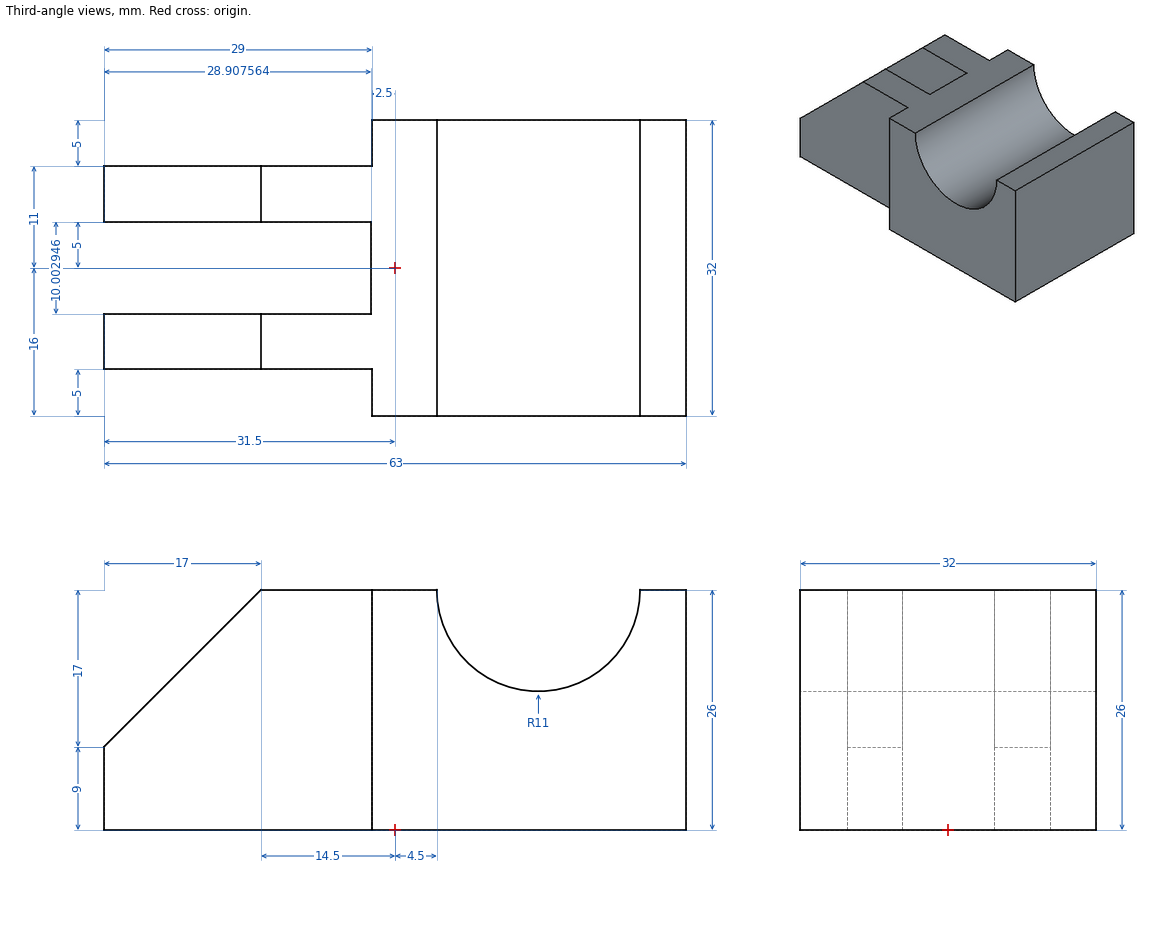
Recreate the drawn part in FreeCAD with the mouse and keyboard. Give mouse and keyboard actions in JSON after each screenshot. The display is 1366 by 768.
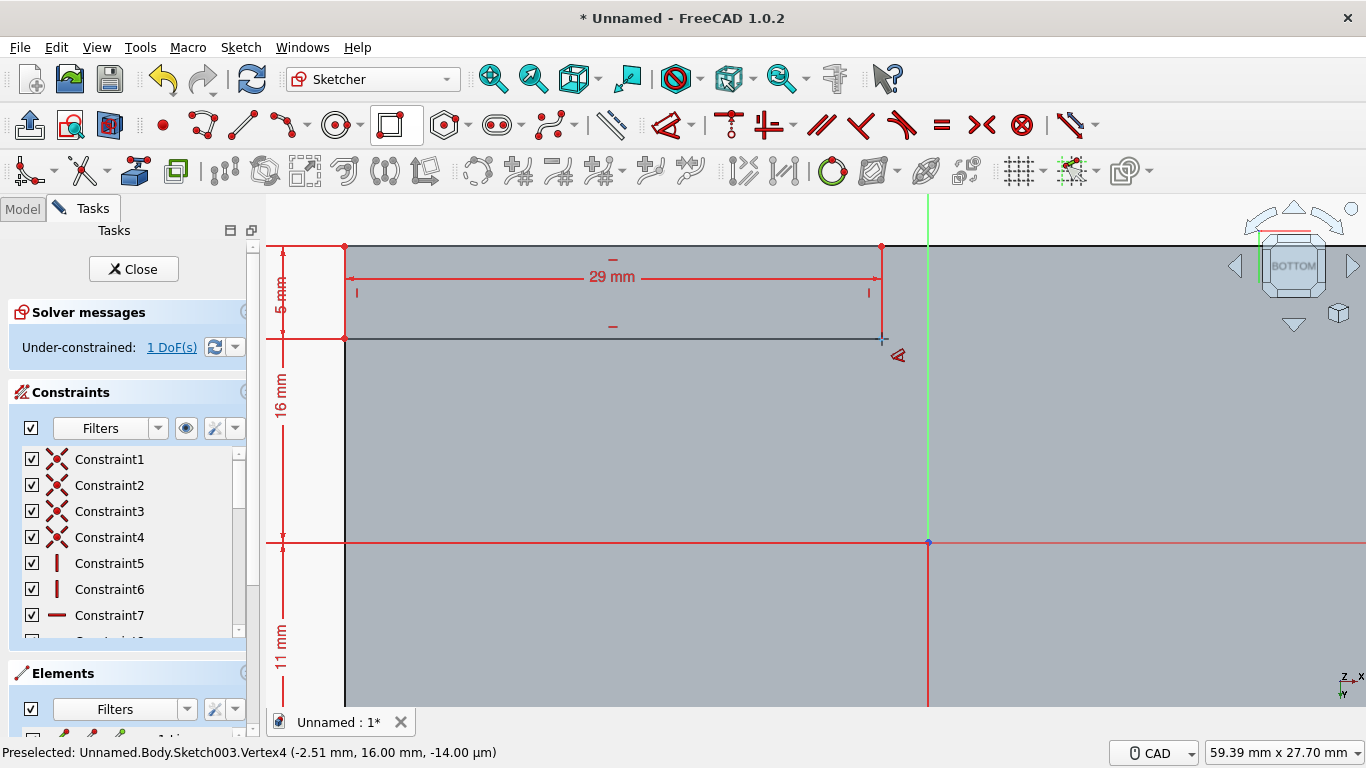
{"action": "left_click", "coordinate": [882, 339]}
{"action": "left_click", "coordinate": [905, 305]}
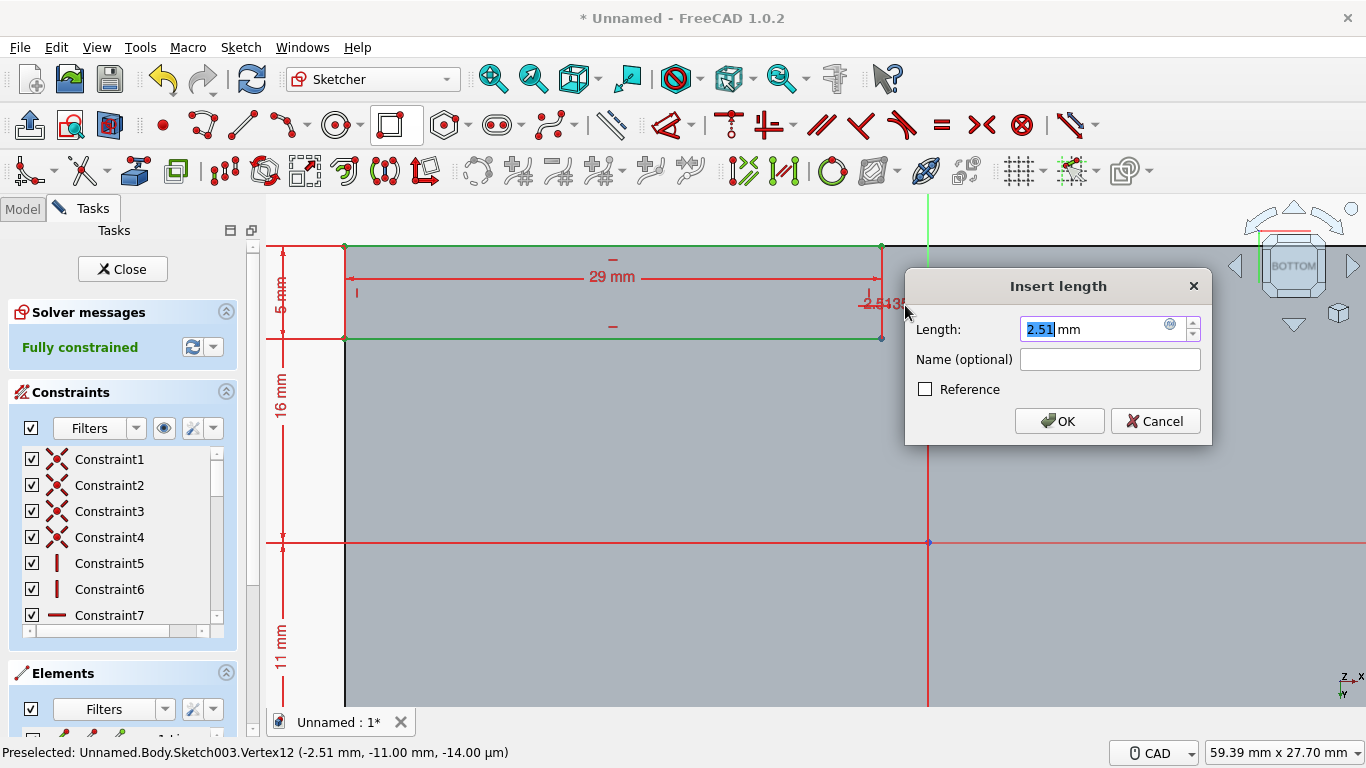
{"action": "type", "text": "2.5"}
{"action": "key", "text": "Return"}
{"action": "key", "text": "Escape"}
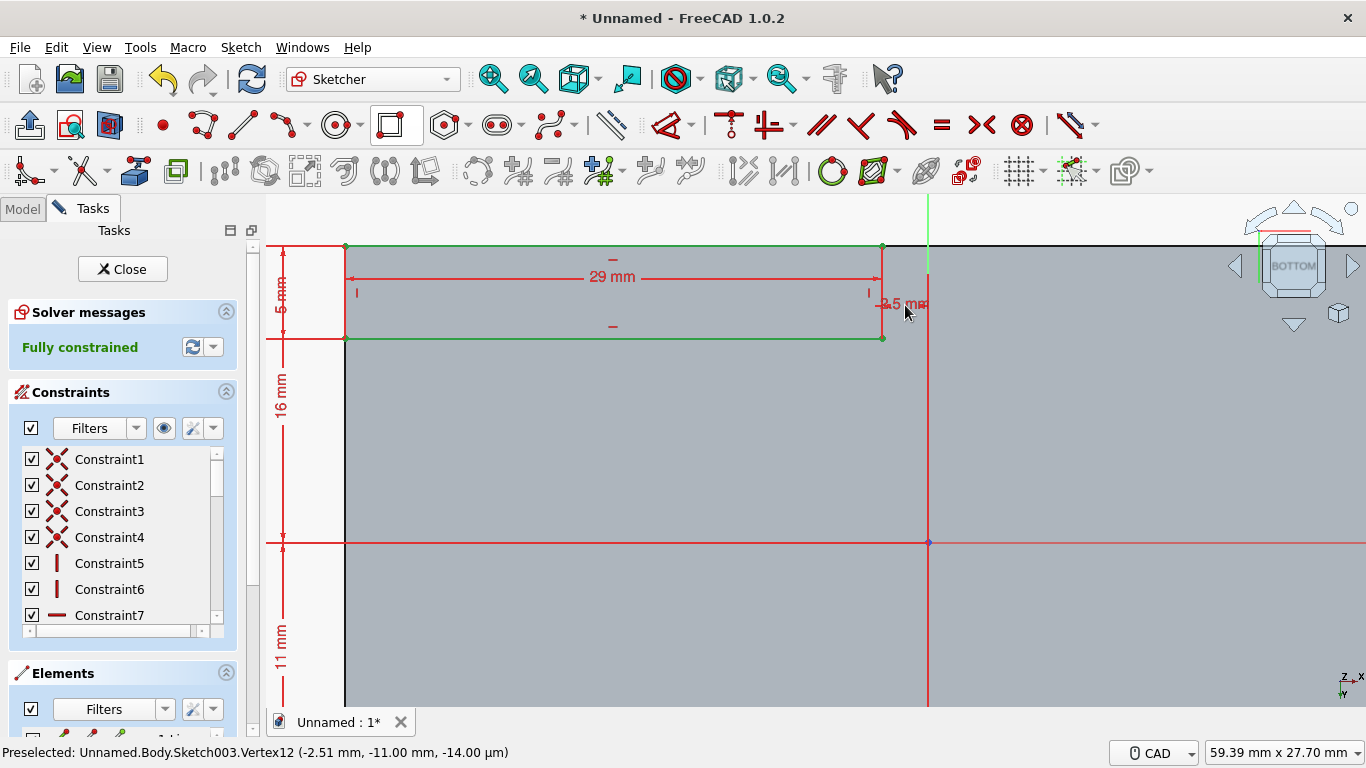
{"action": "left_click", "coordinate": [123, 269]}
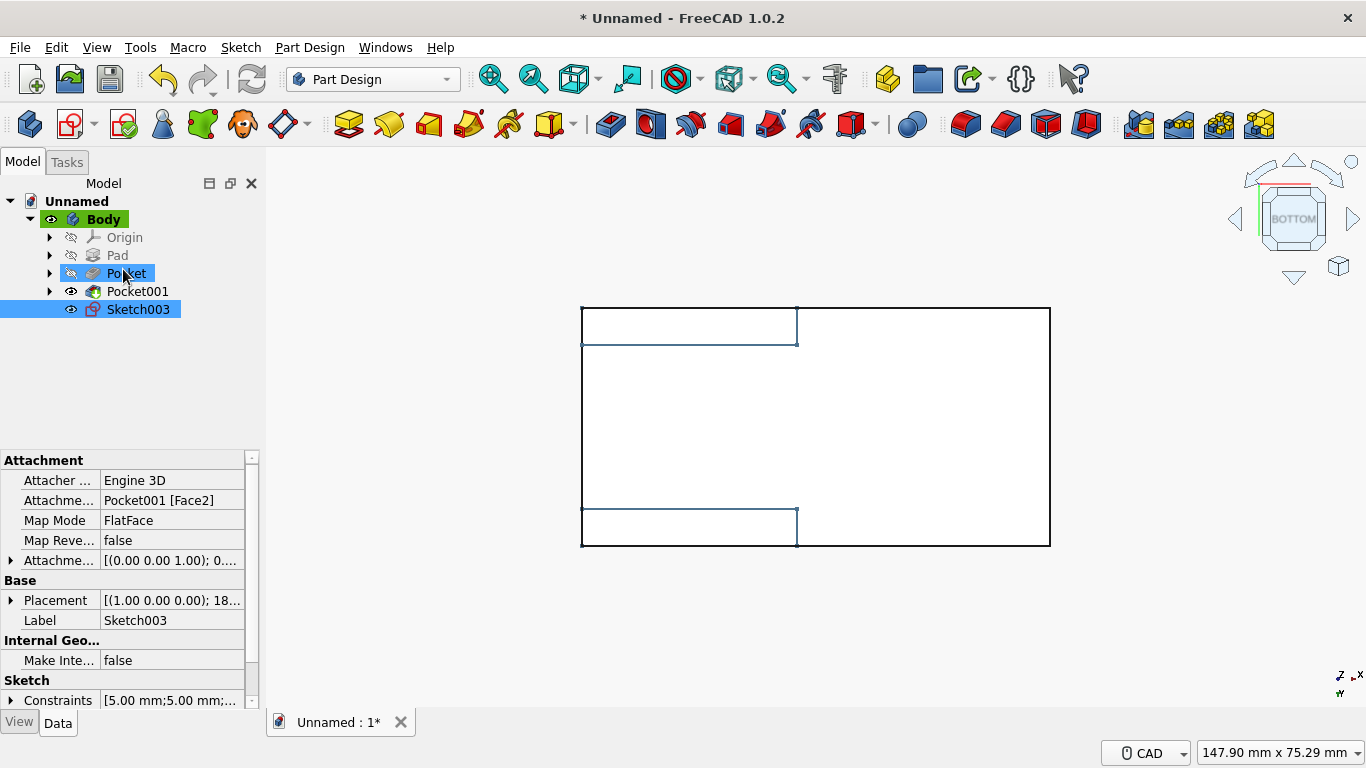
{"action": "left_click", "coordinate": [612, 124]}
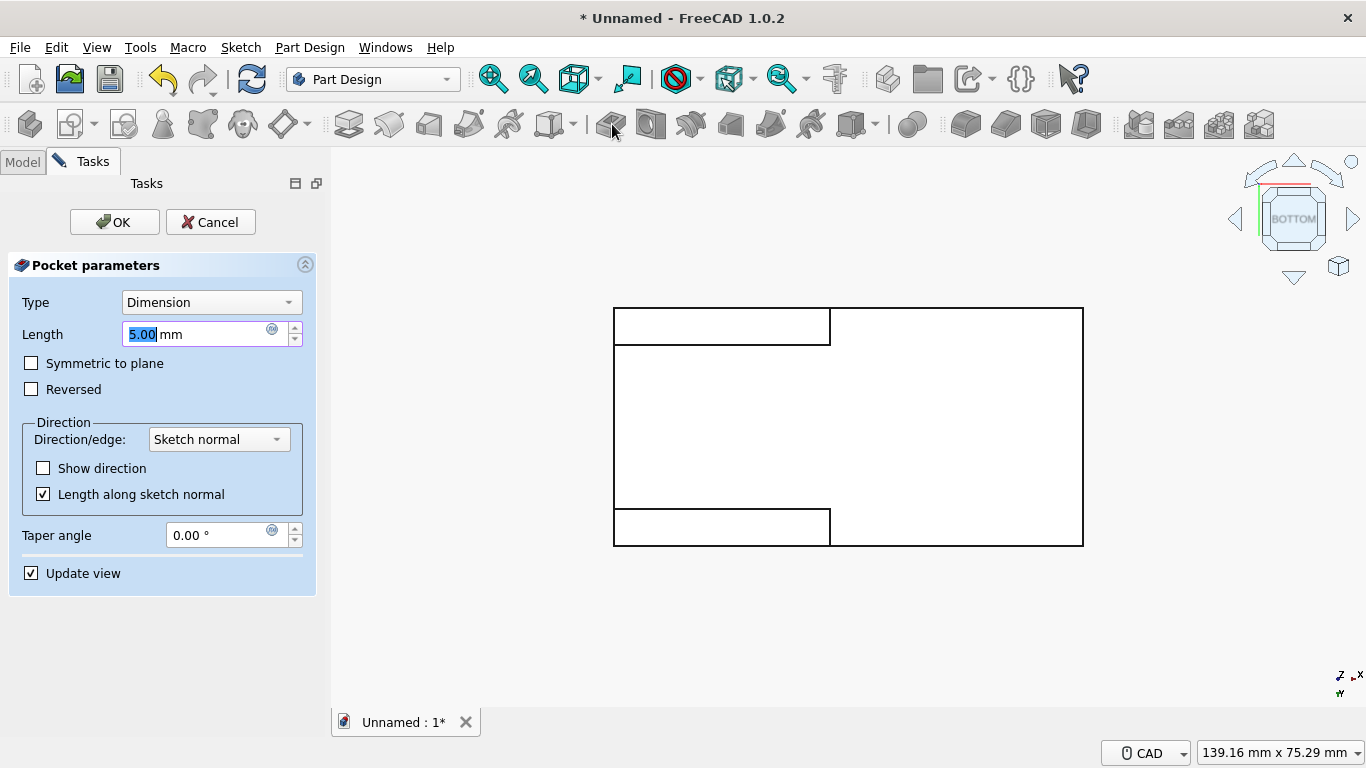
{"action": "left_click", "coordinate": [212, 302]}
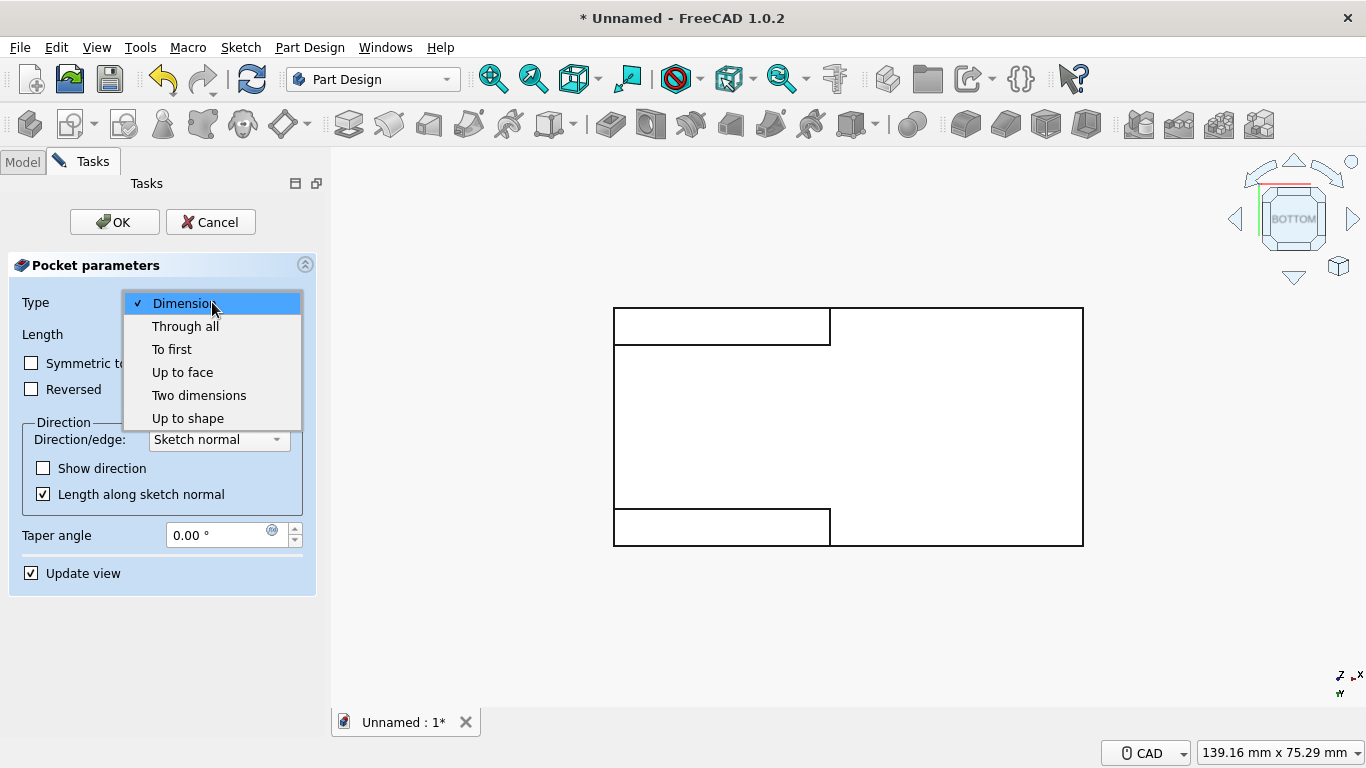
{"action": "left_click", "coordinate": [212, 326]}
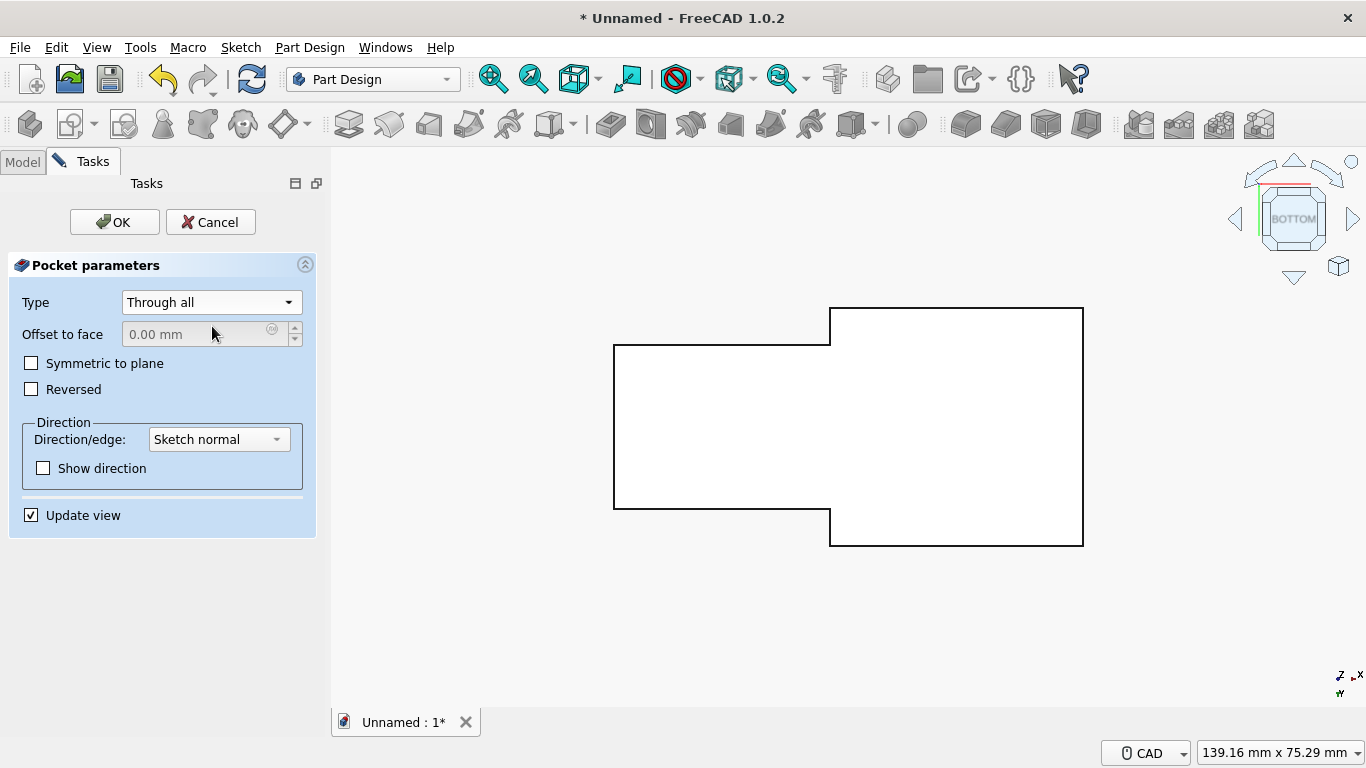
{"action": "left_click", "coordinate": [115, 222]}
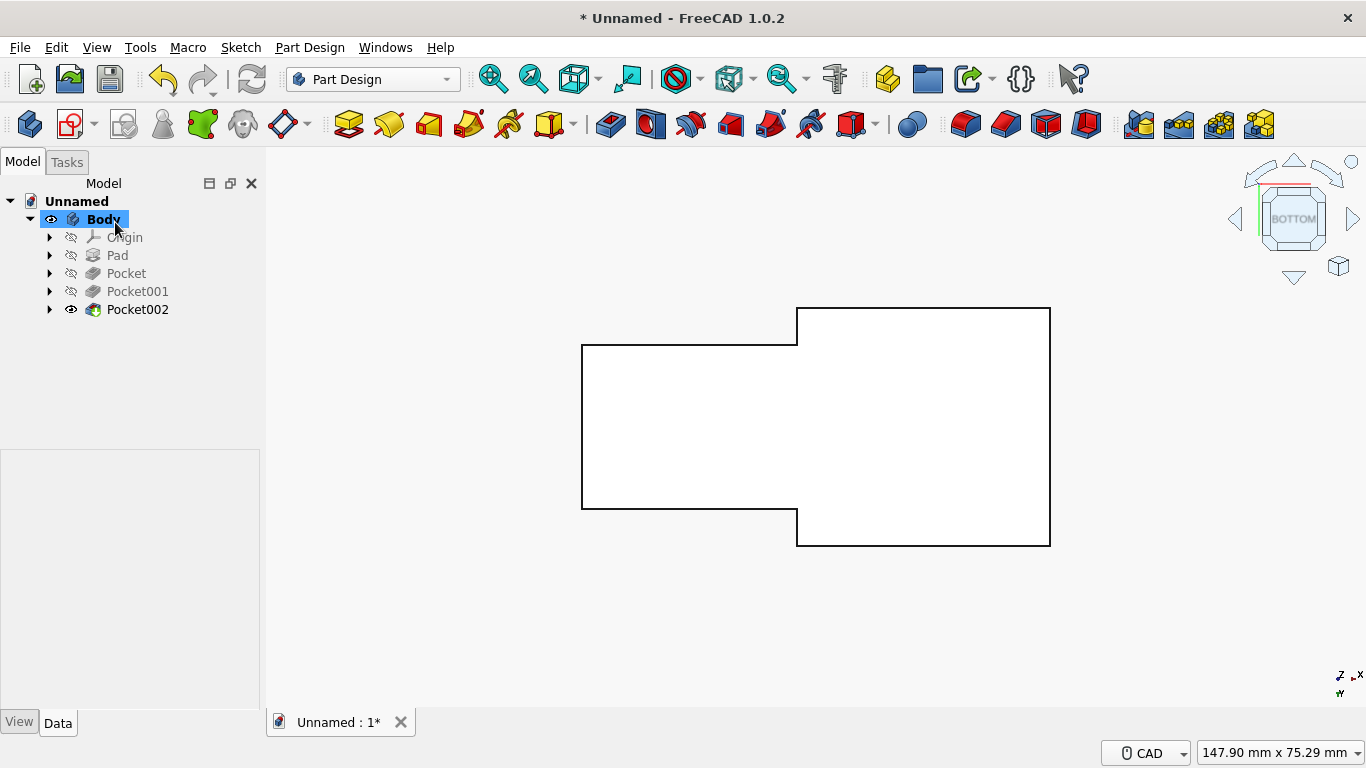
{"action": "left_click", "coordinate": [494, 80]}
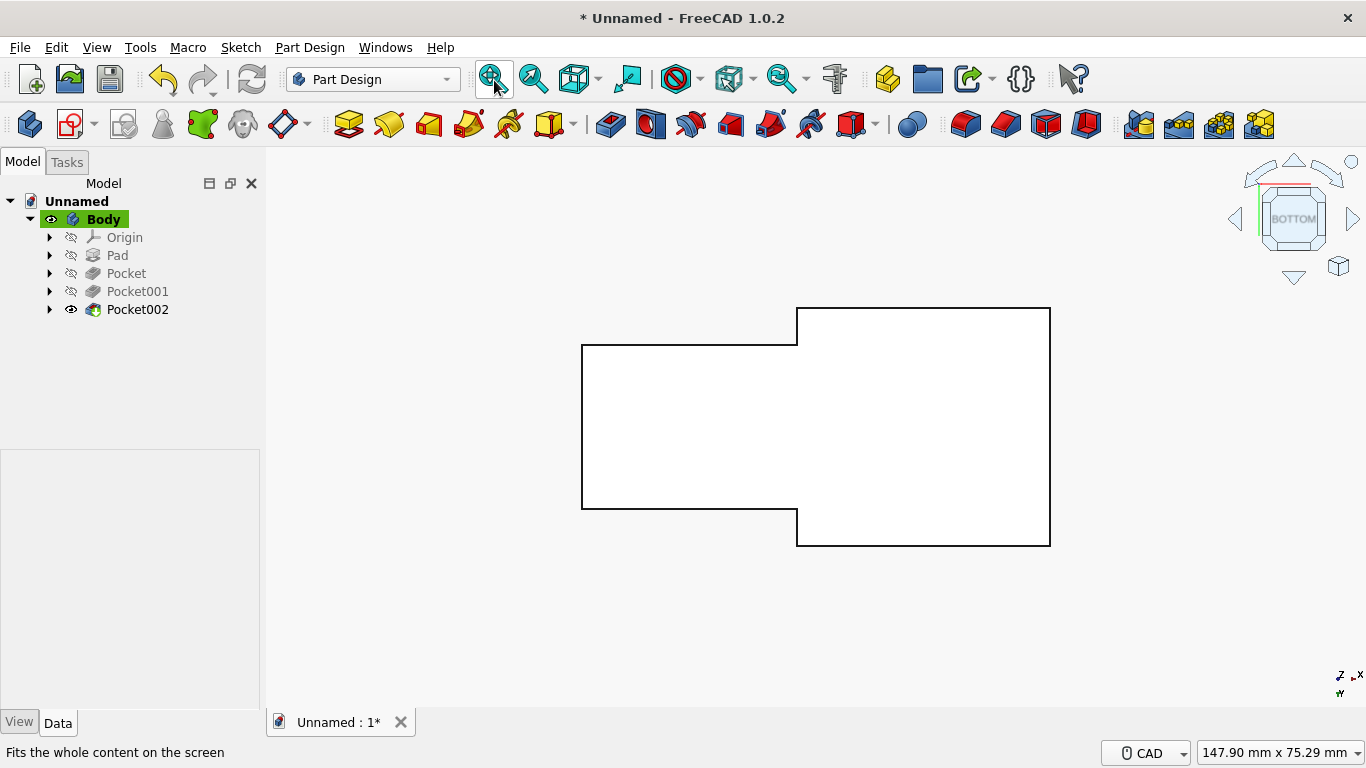
{"action": "left_click", "coordinate": [883, 426]}